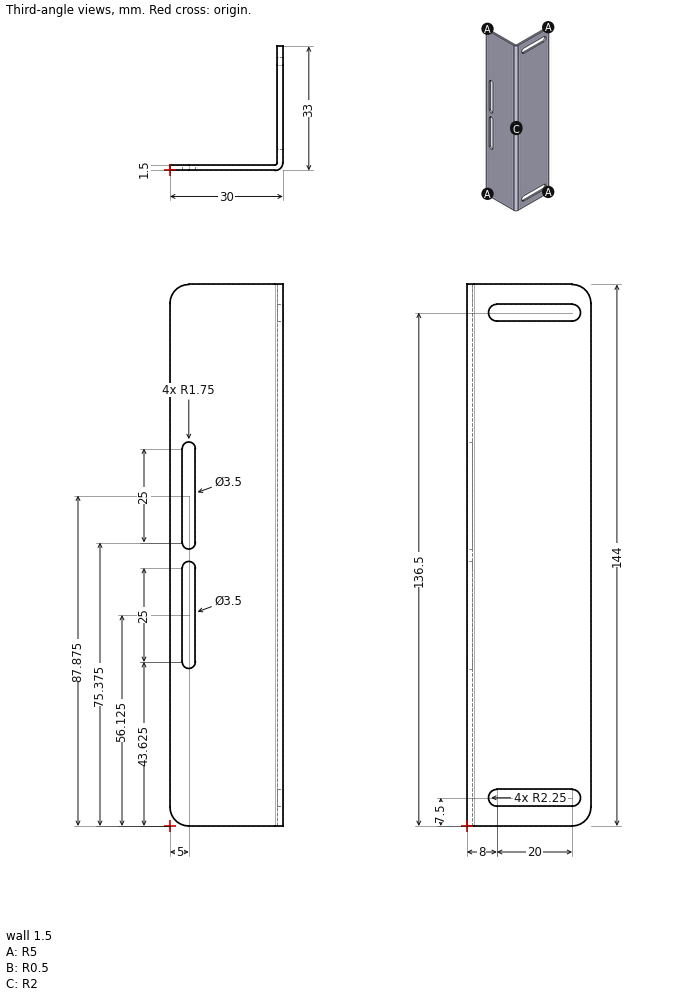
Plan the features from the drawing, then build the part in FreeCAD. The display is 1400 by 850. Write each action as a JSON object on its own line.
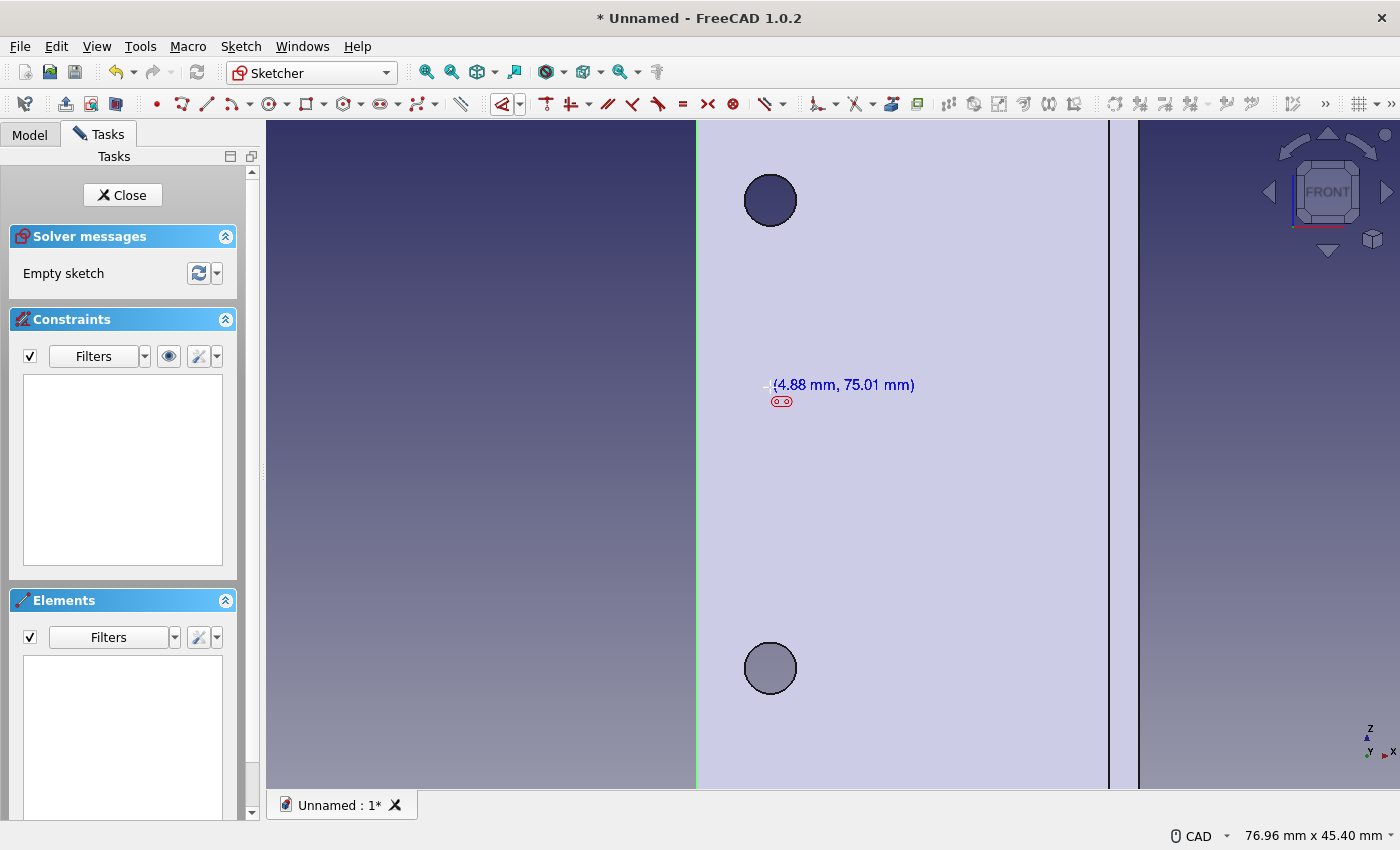
{"action": "scroll", "coordinate": [772, 330], "scroll_direction": "down", "scroll_amount": 6}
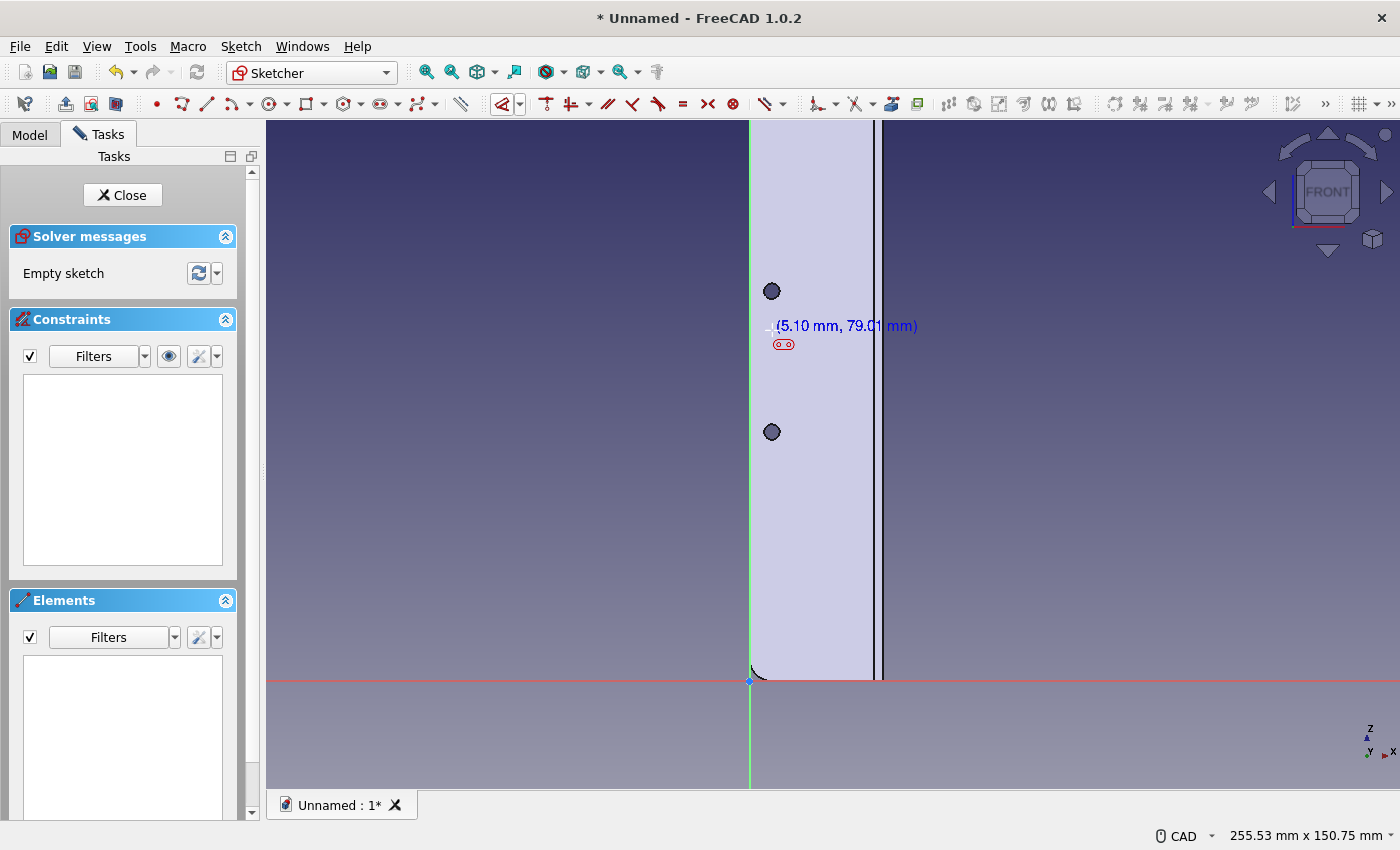
{"action": "left_click", "coordinate": [772, 347]}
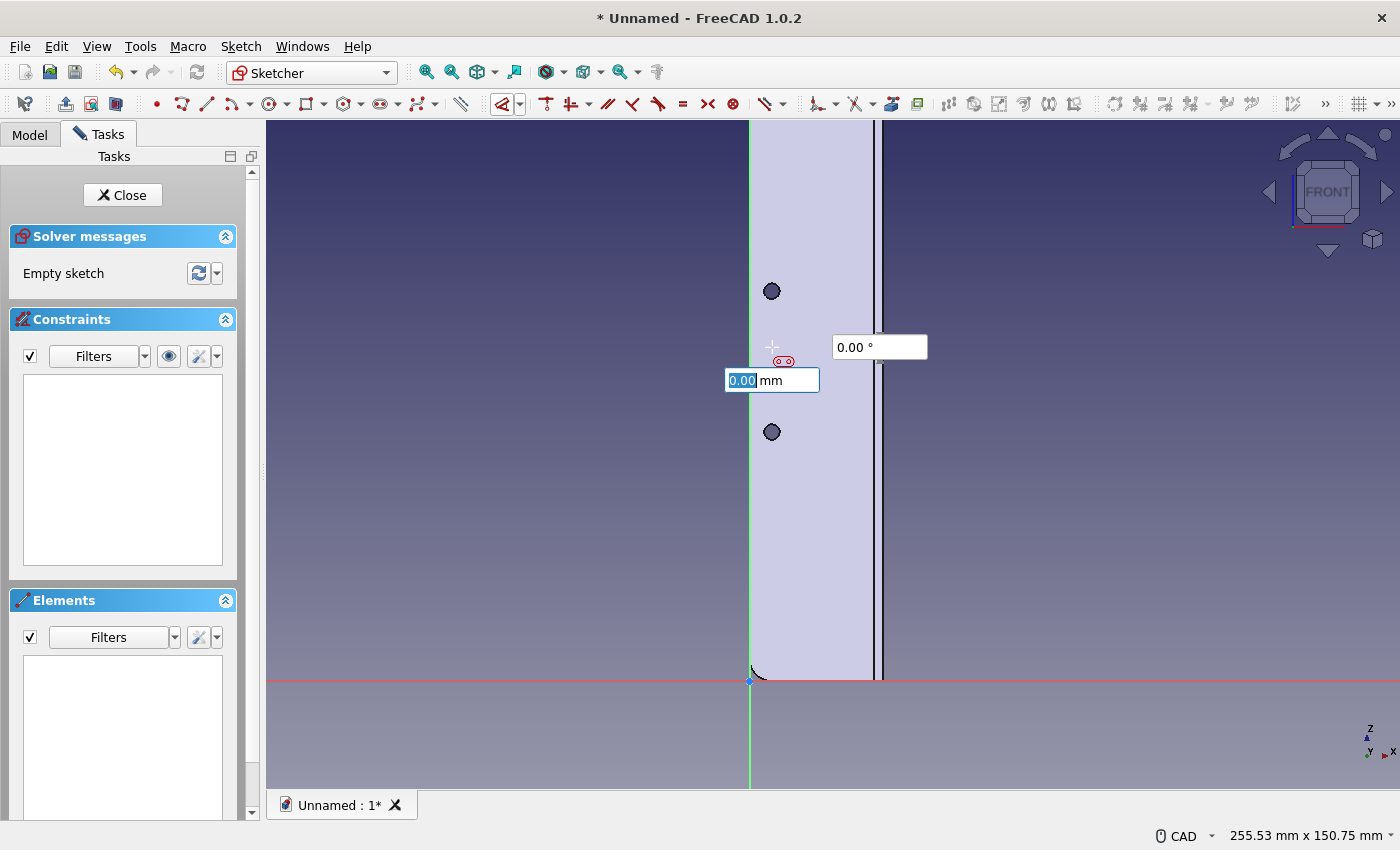
{"action": "left_click", "coordinate": [772, 236]}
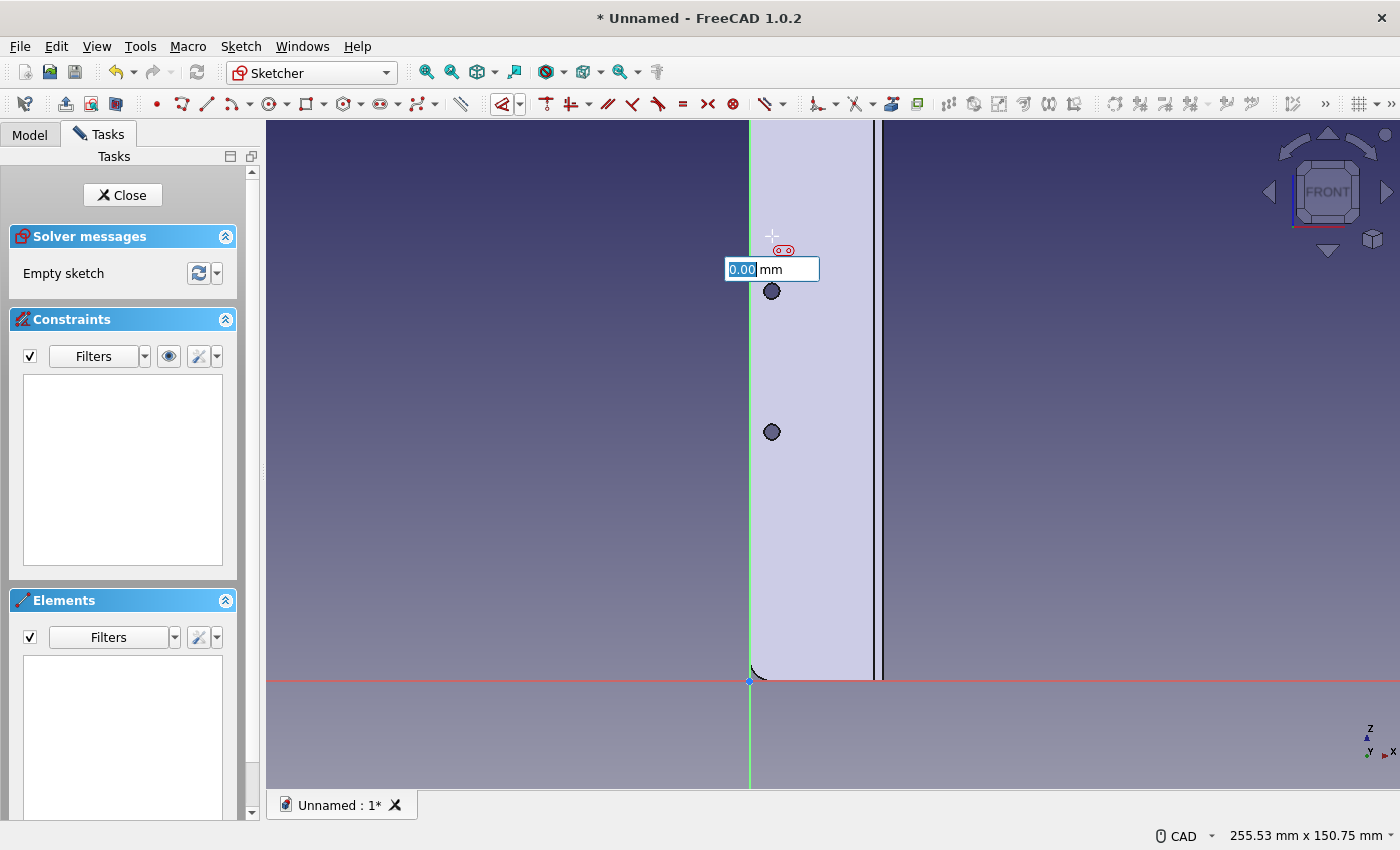
{"action": "scroll", "coordinate": [764, 291], "scroll_direction": "up", "scroll_amount": 4}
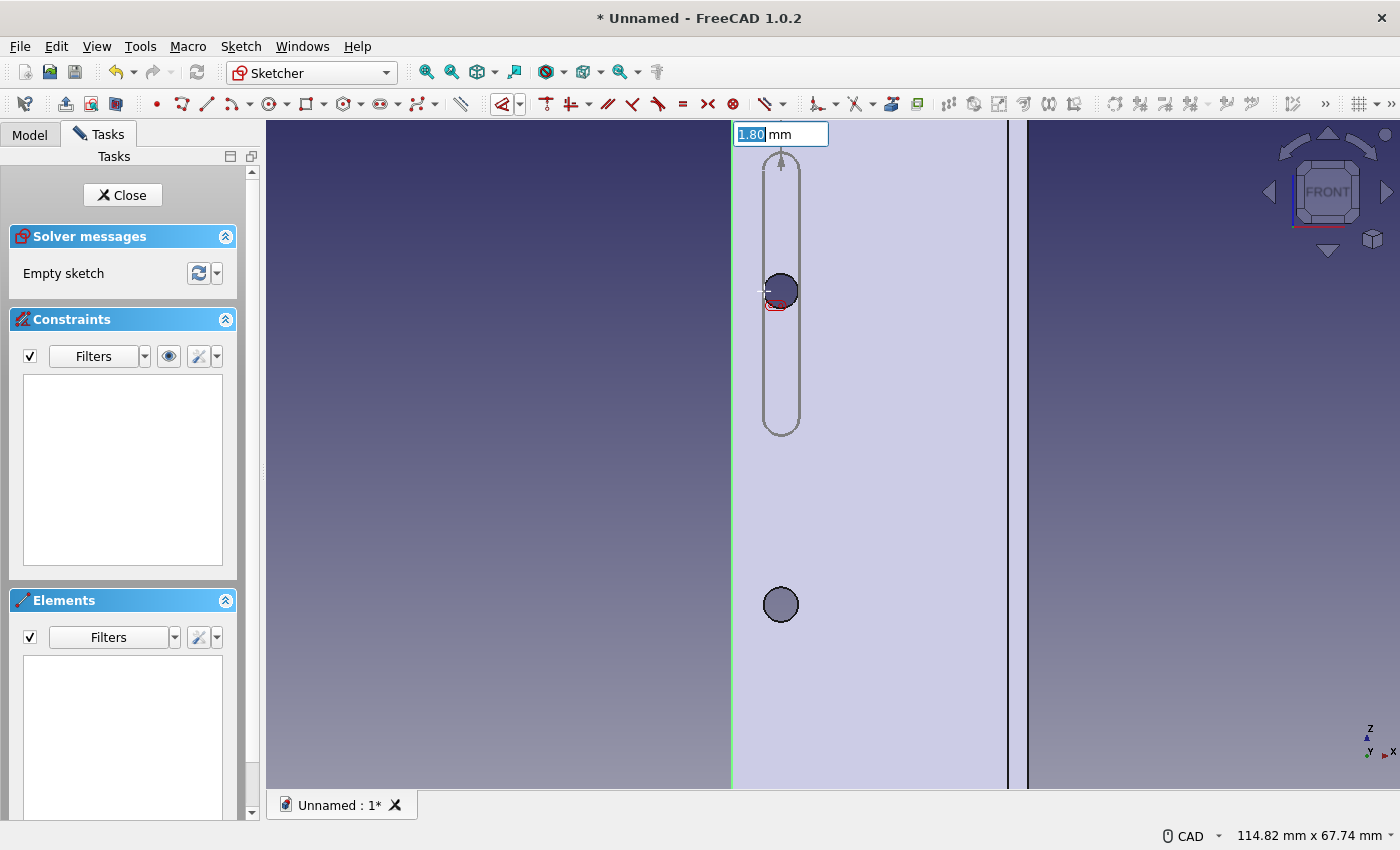
{"action": "left_click", "coordinate": [764, 291]}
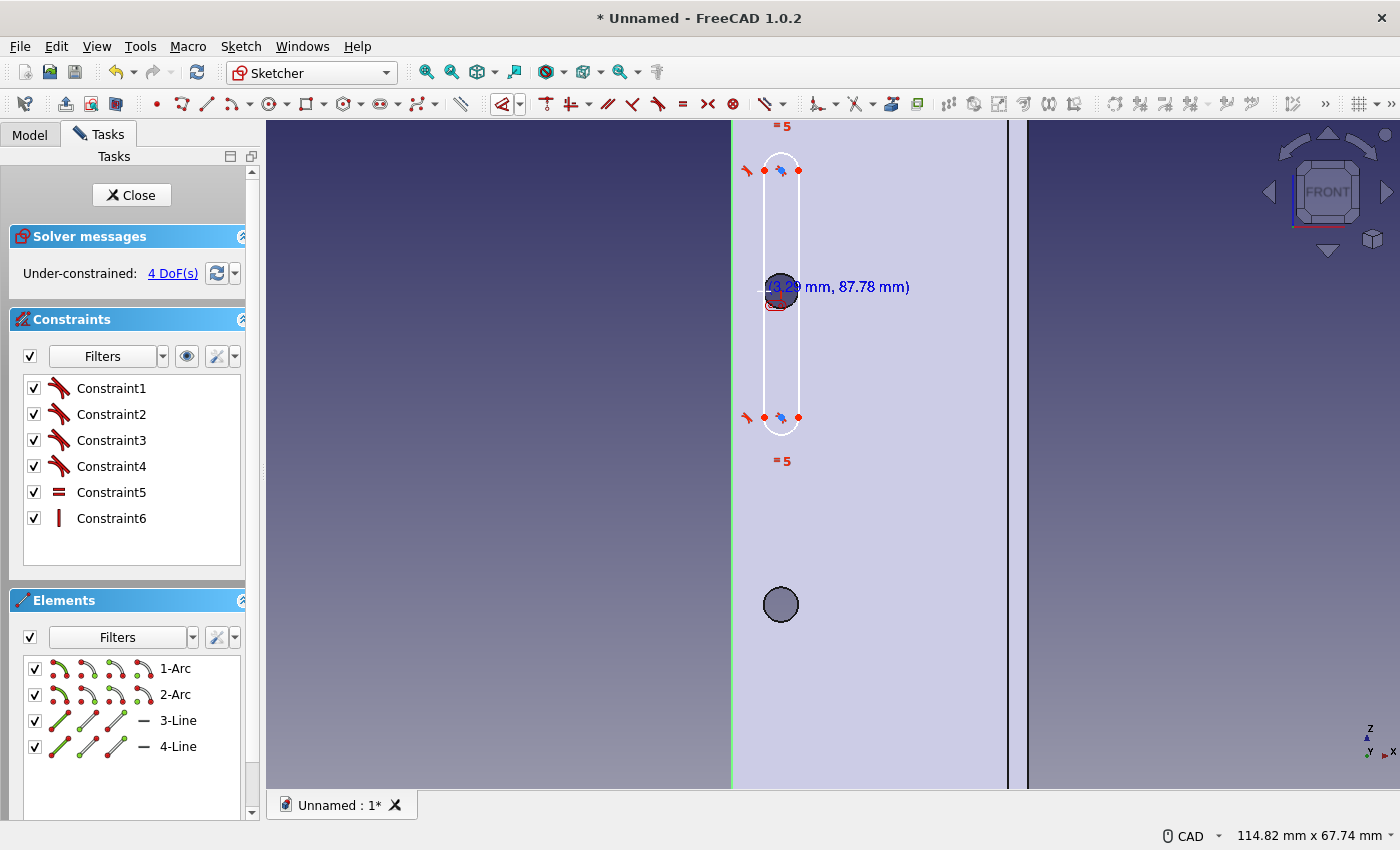
{"action": "scroll", "coordinate": [781, 728], "scroll_direction": "up", "scroll_amount": 2}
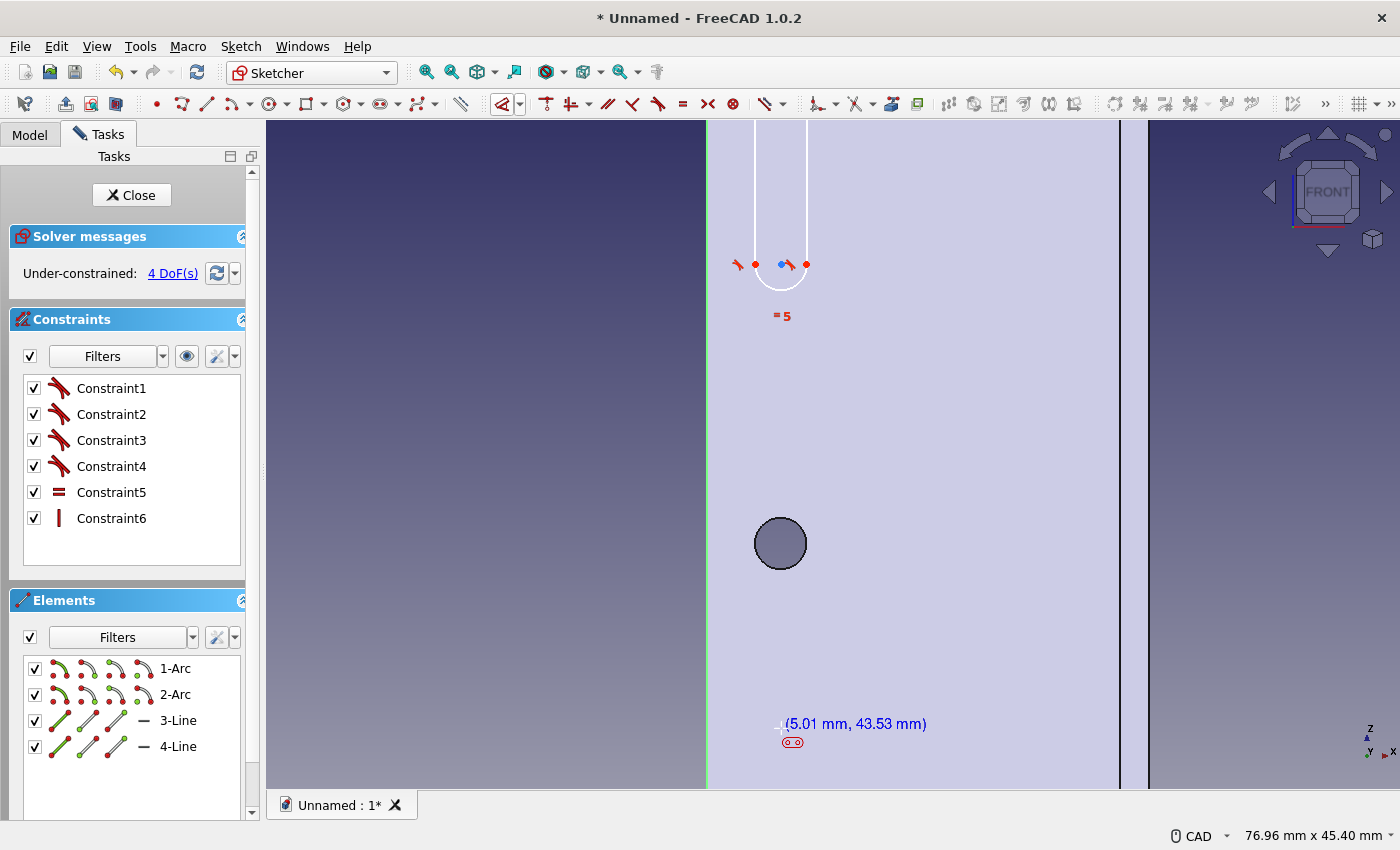
{"action": "scroll", "coordinate": [768, 384], "scroll_direction": "down", "scroll_amount": 6}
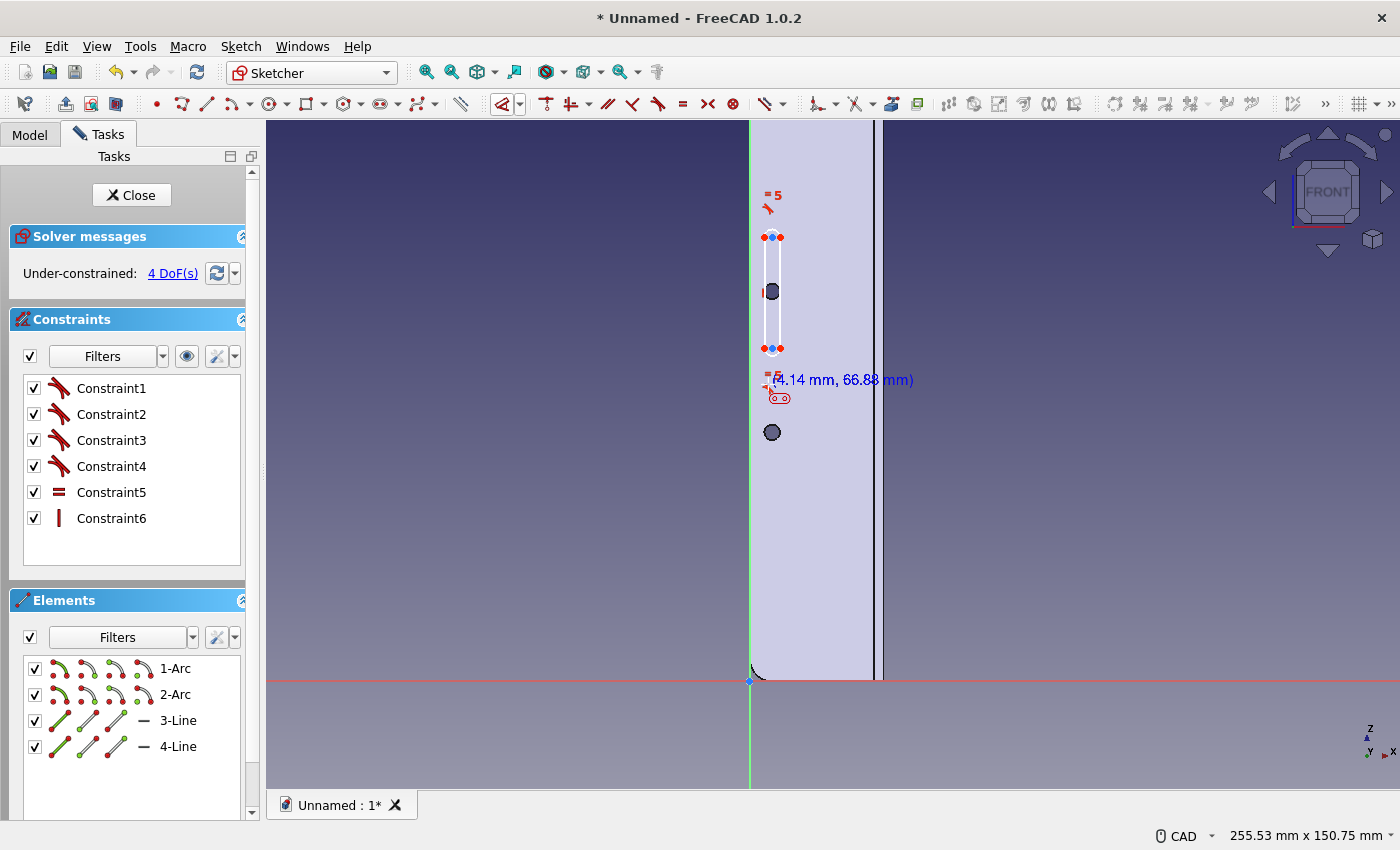
{"action": "left_click", "coordinate": [772, 488]}